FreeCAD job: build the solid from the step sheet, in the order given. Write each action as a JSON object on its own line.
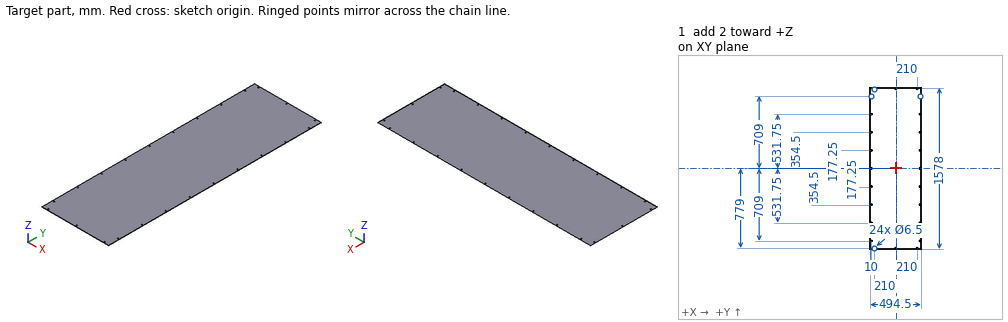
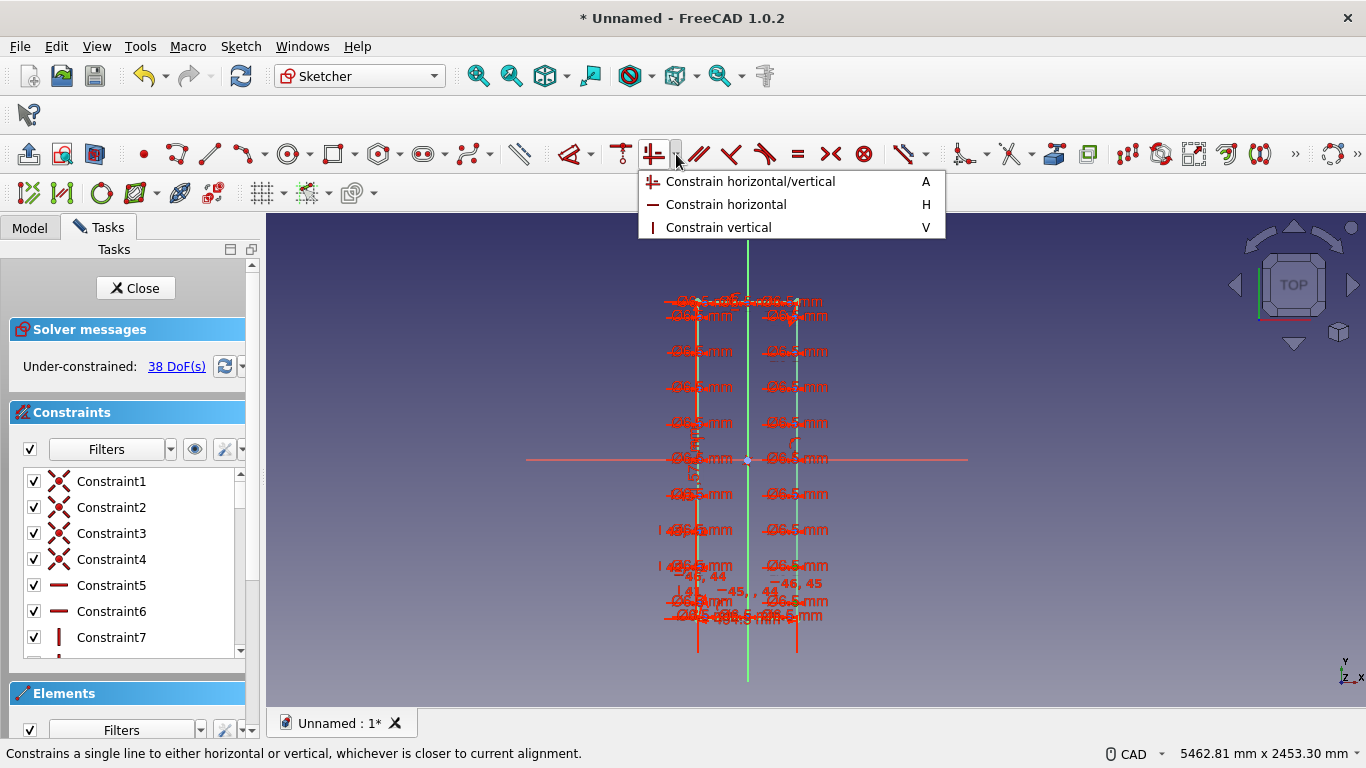
{"action": "left_click", "coordinate": [792, 228]}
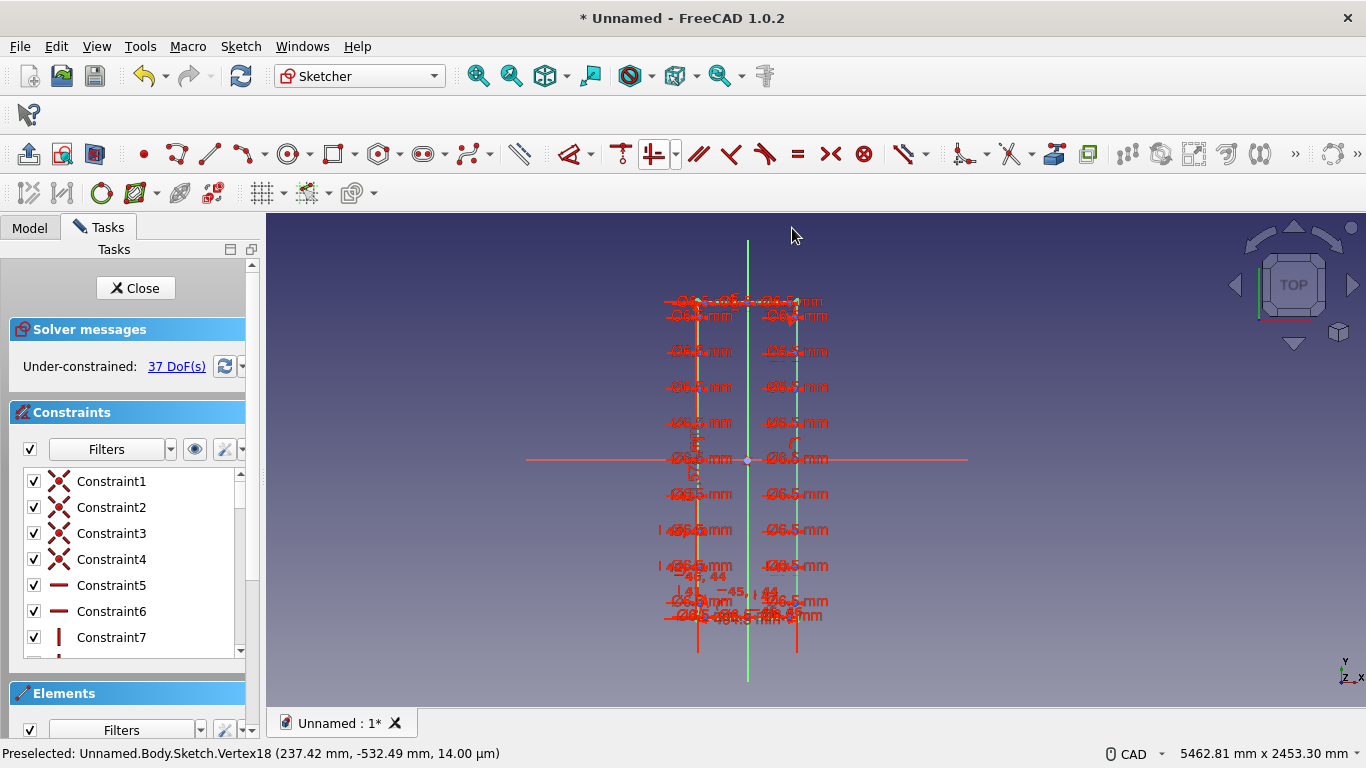
{"action": "left_click", "coordinate": [700, 568]}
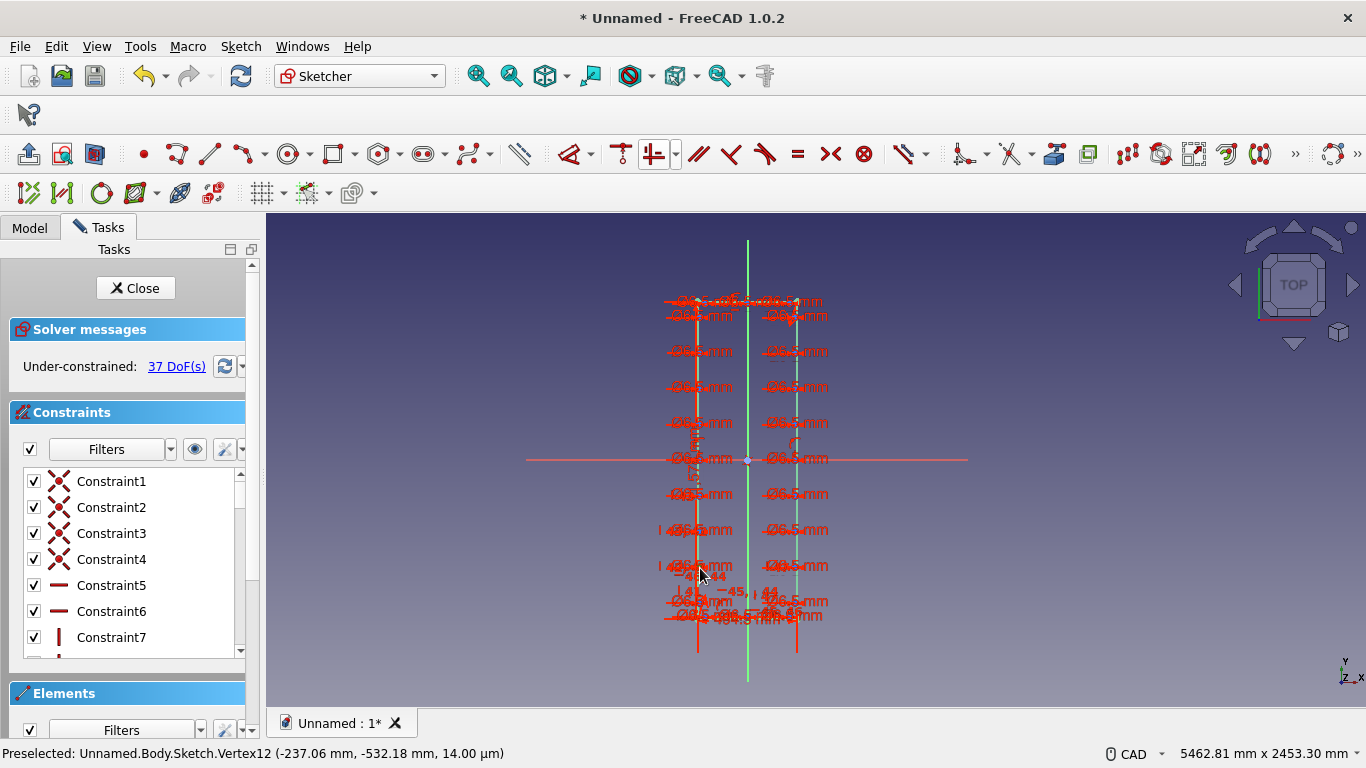
{"action": "left_click", "coordinate": [795, 568]}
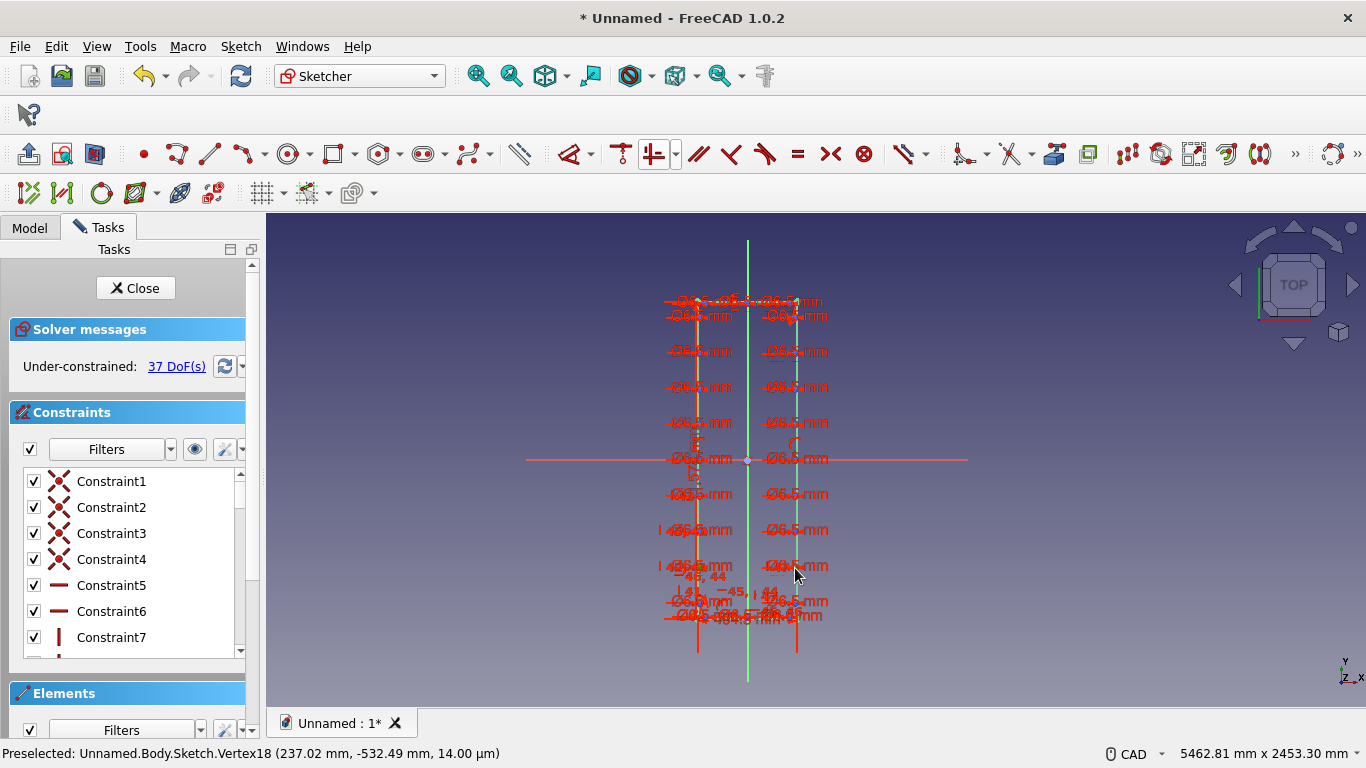
{"action": "key", "text": "h"}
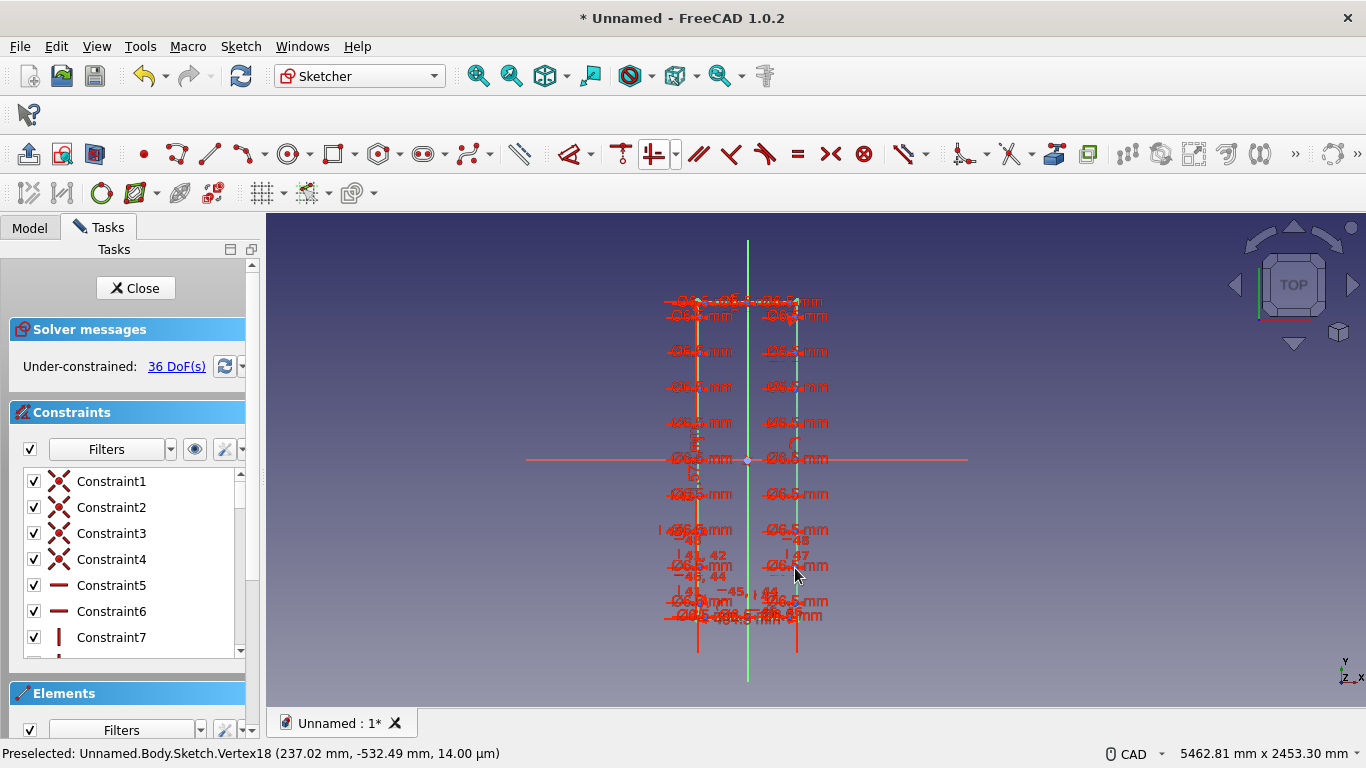
{"action": "left_click", "coordinate": [795, 568]}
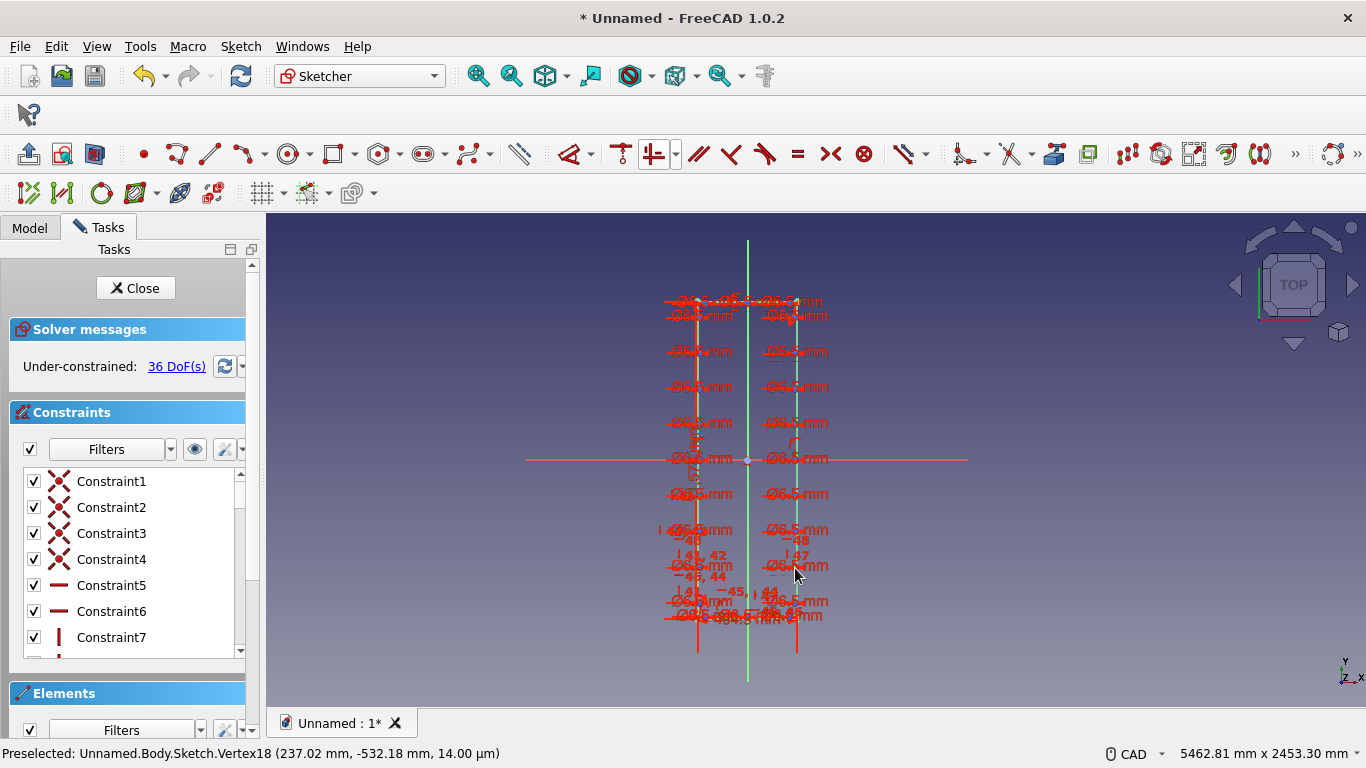
{"action": "left_click", "coordinate": [793, 530]}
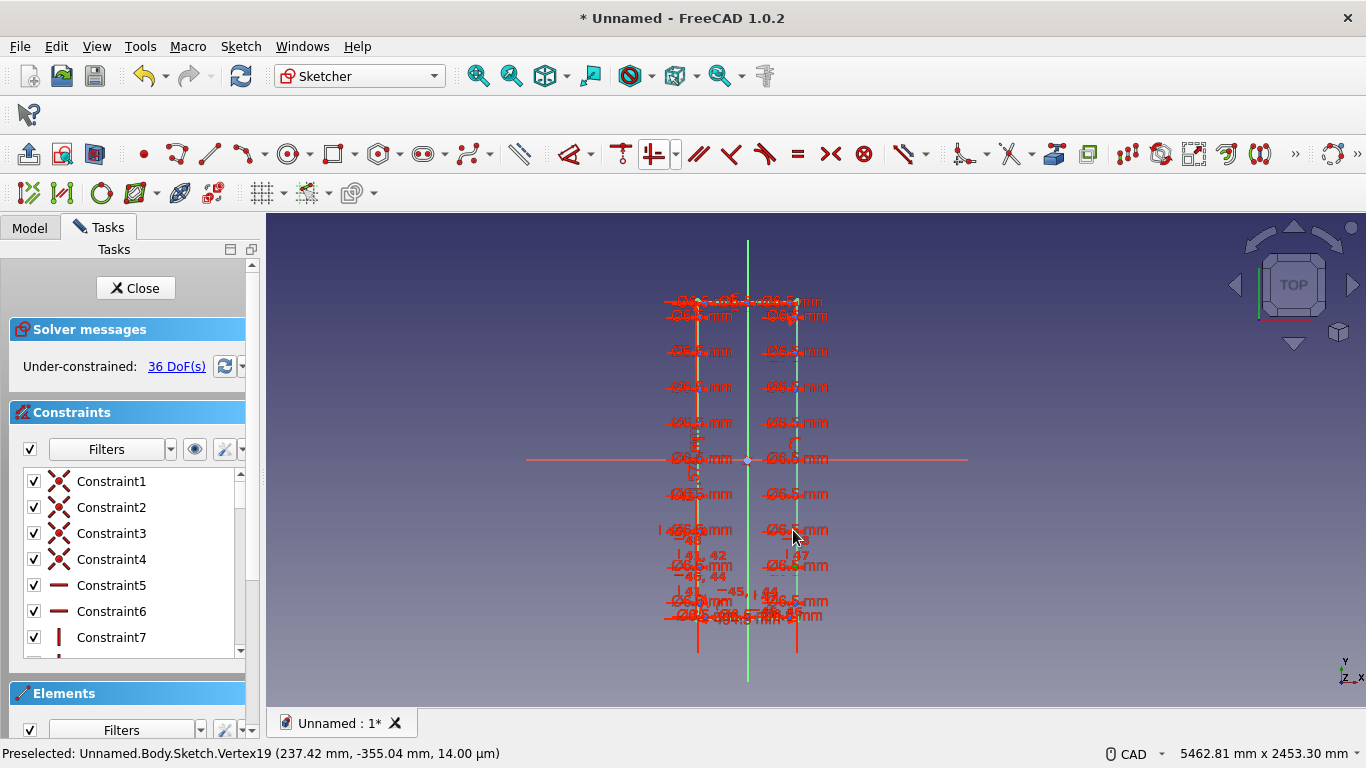
{"action": "key", "text": "v"}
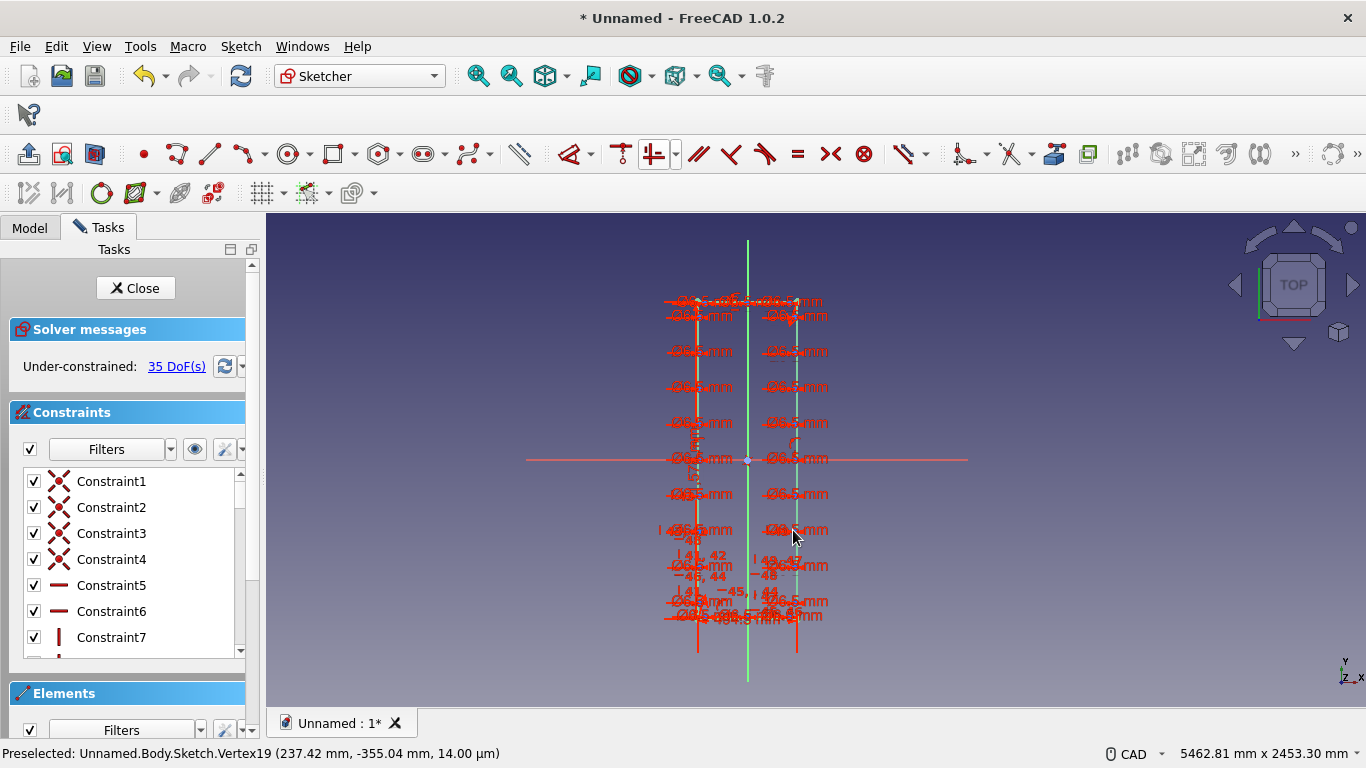
{"action": "left_click", "coordinate": [700, 532]}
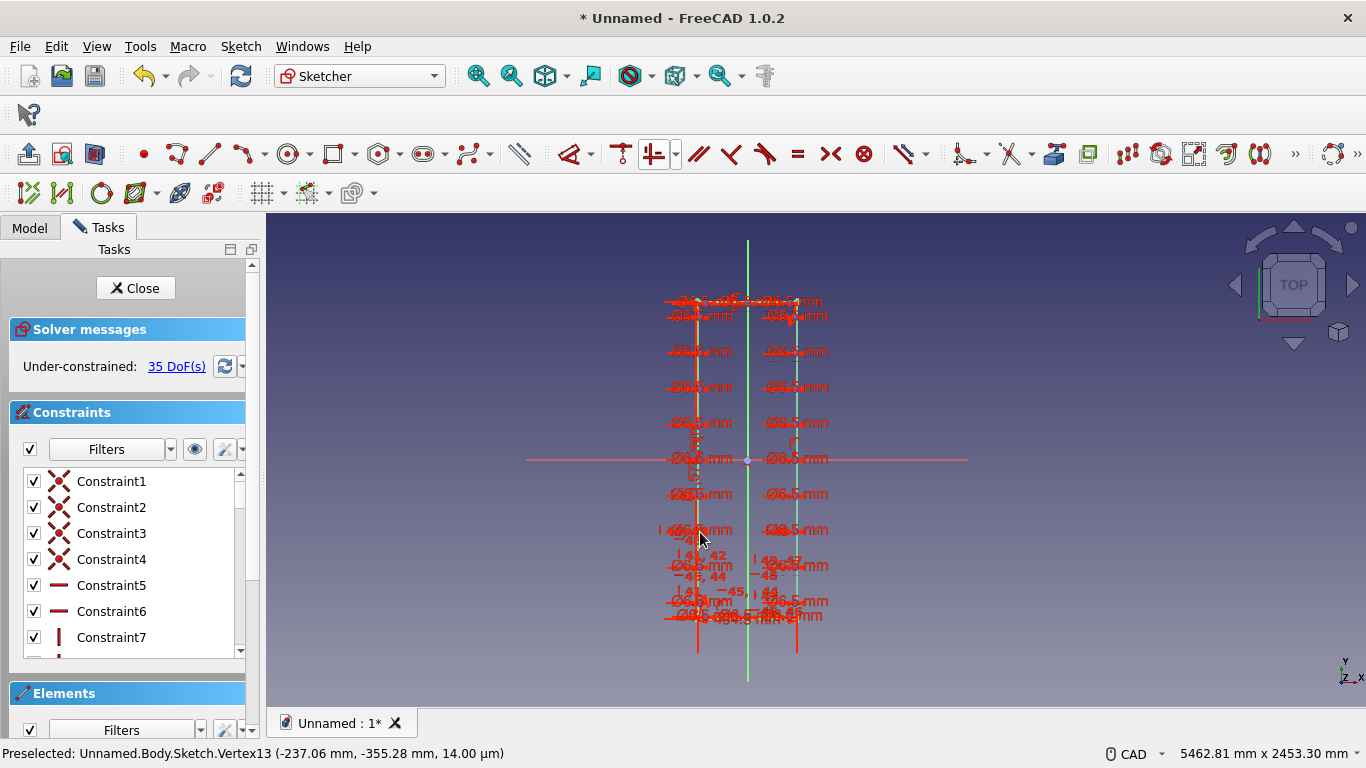
{"action": "left_click", "coordinate": [795, 532]}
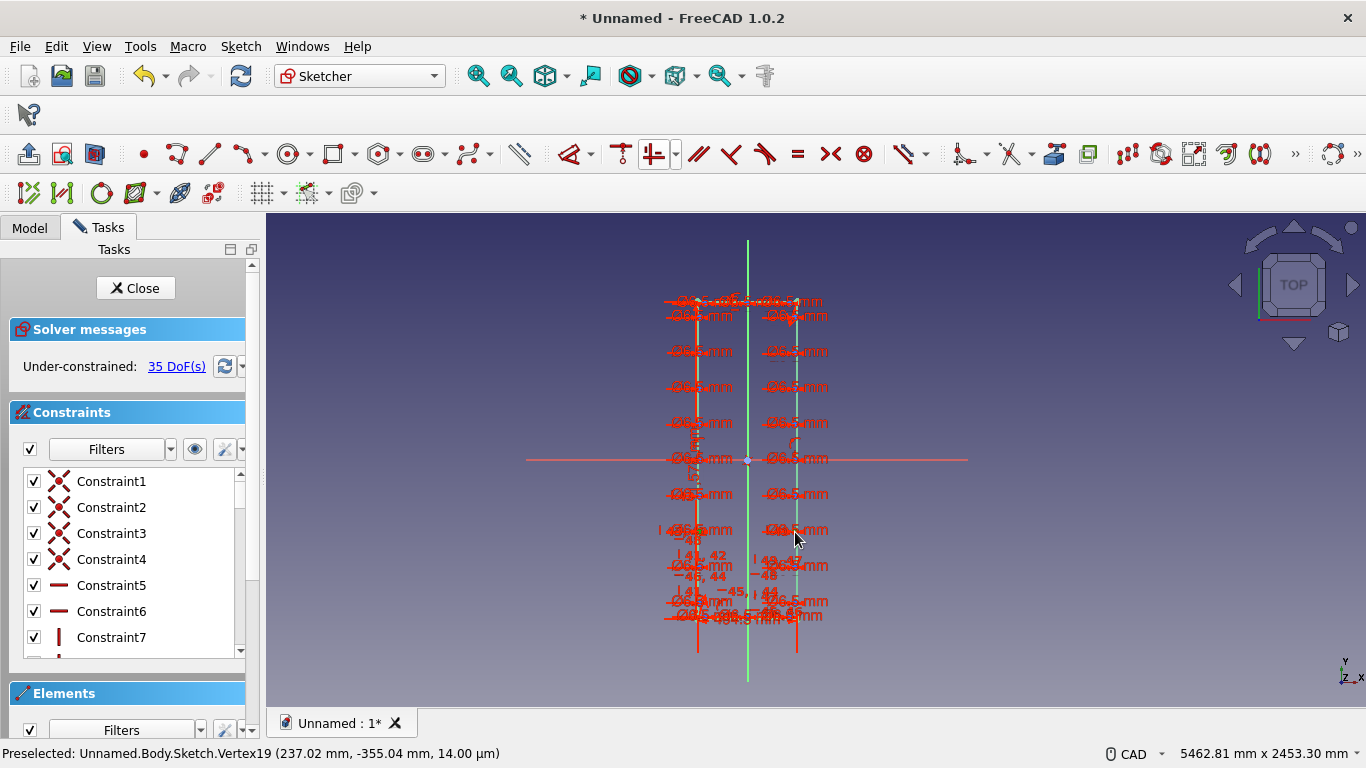
{"action": "key", "text": "h"}